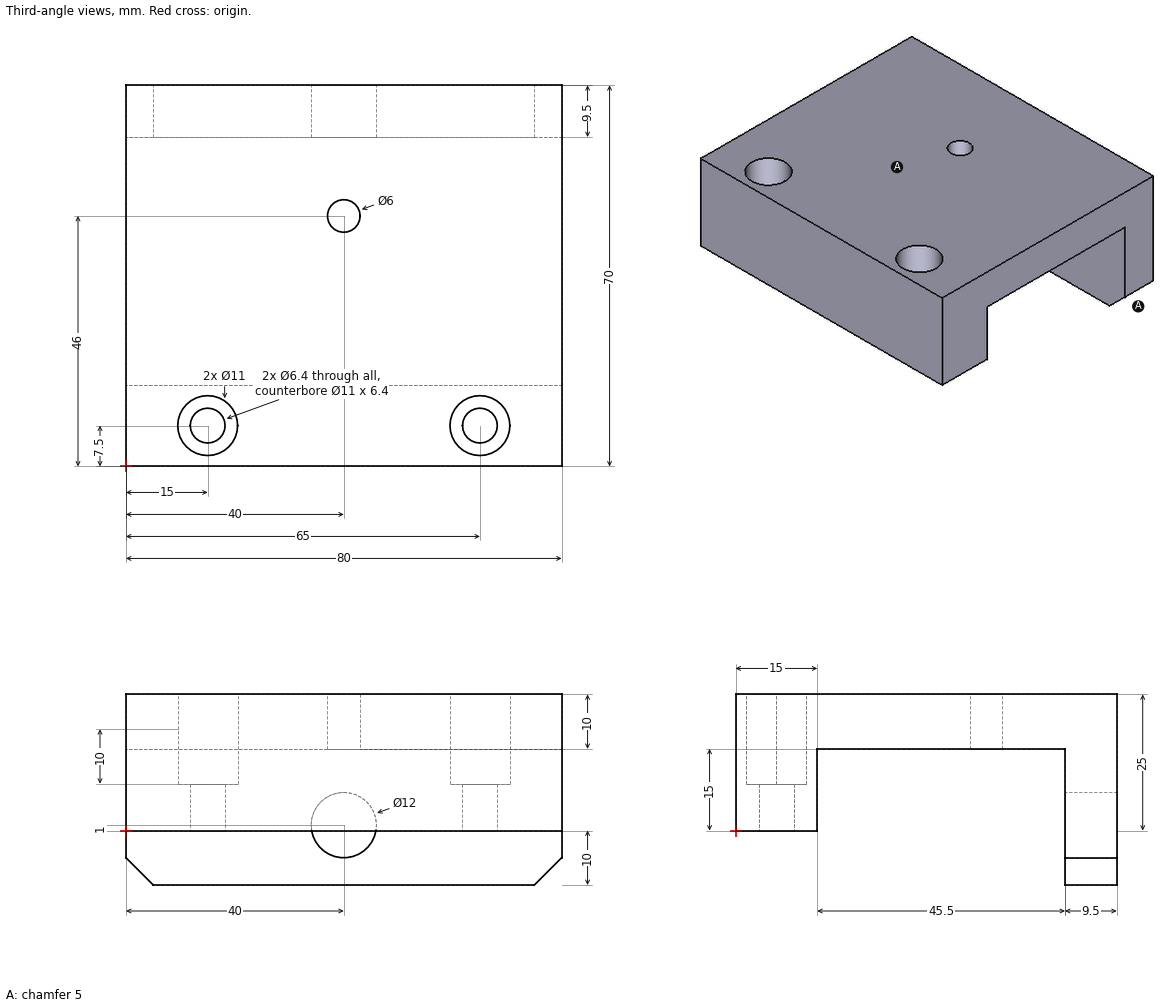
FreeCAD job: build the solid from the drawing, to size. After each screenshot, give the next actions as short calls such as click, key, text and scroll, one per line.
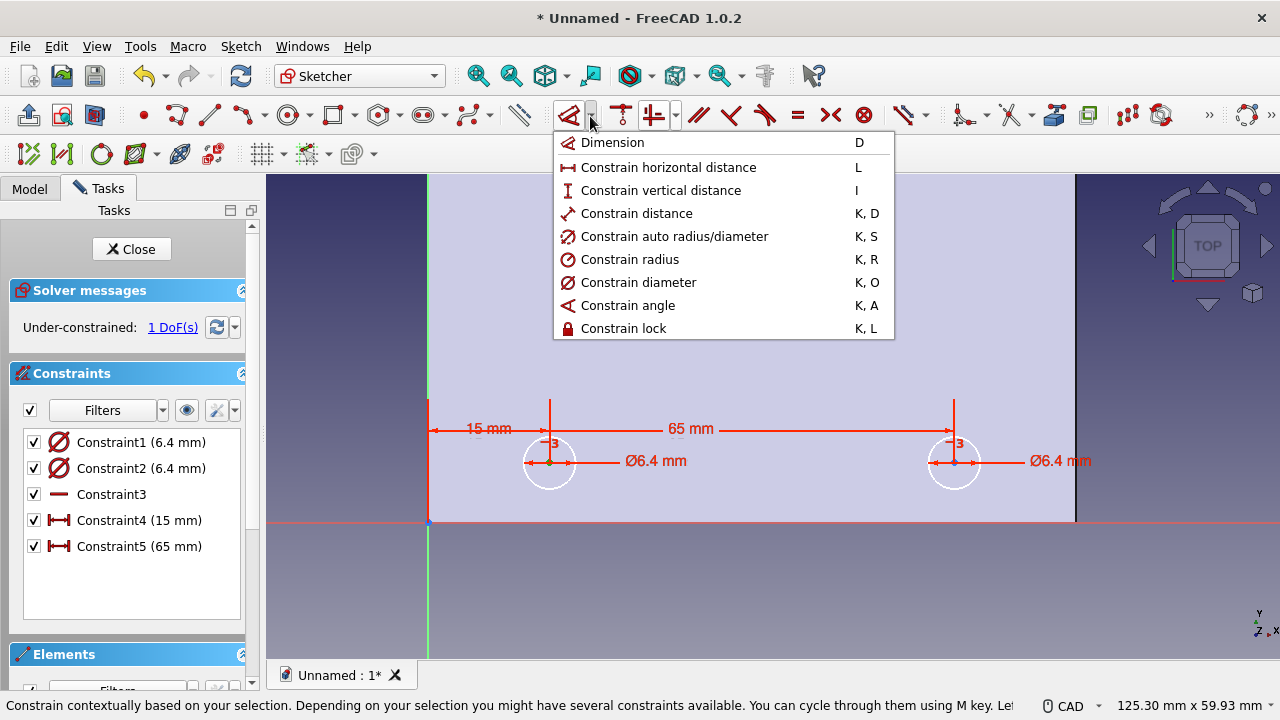
click(724, 190)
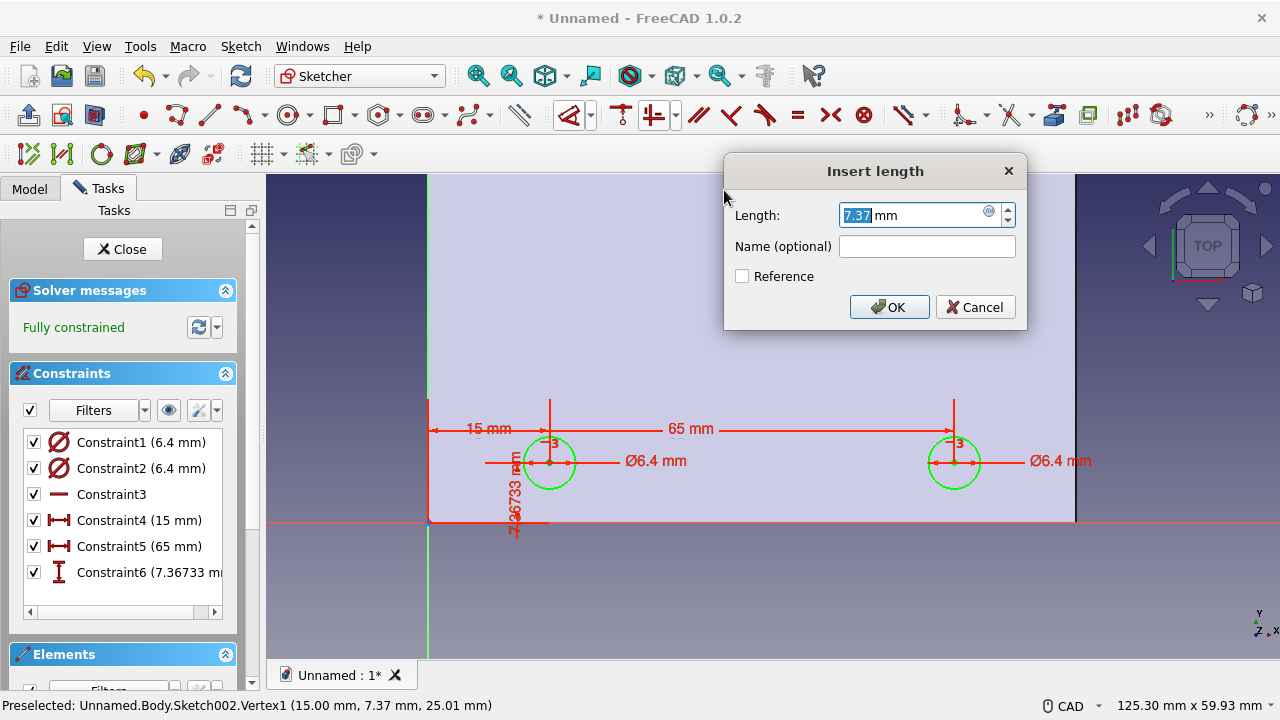
text(7.5)
key(Return)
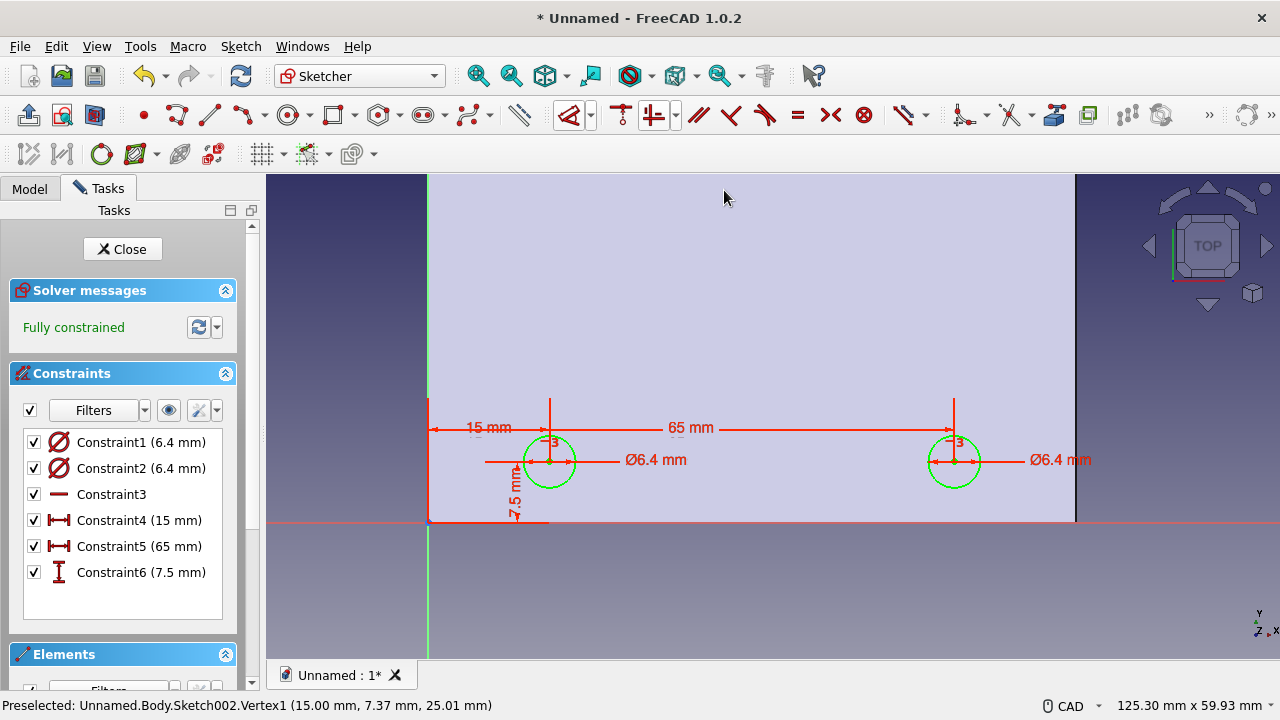
click(123, 249)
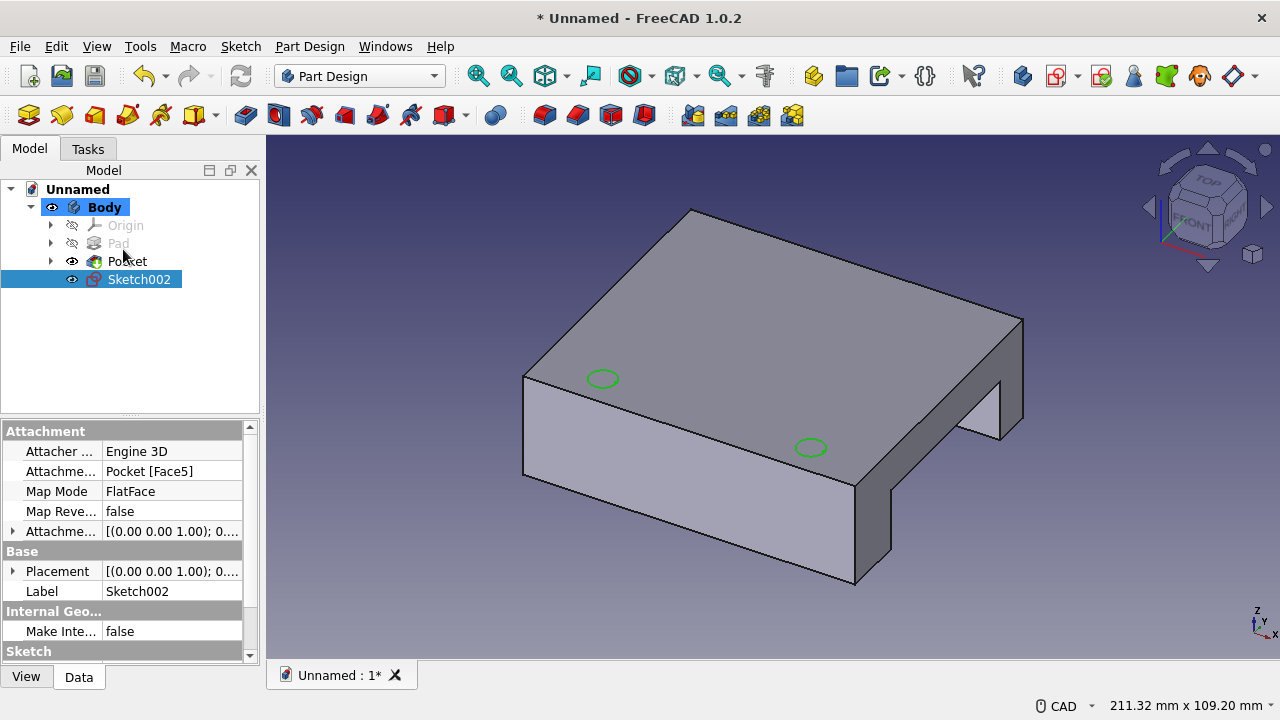
click(279, 116)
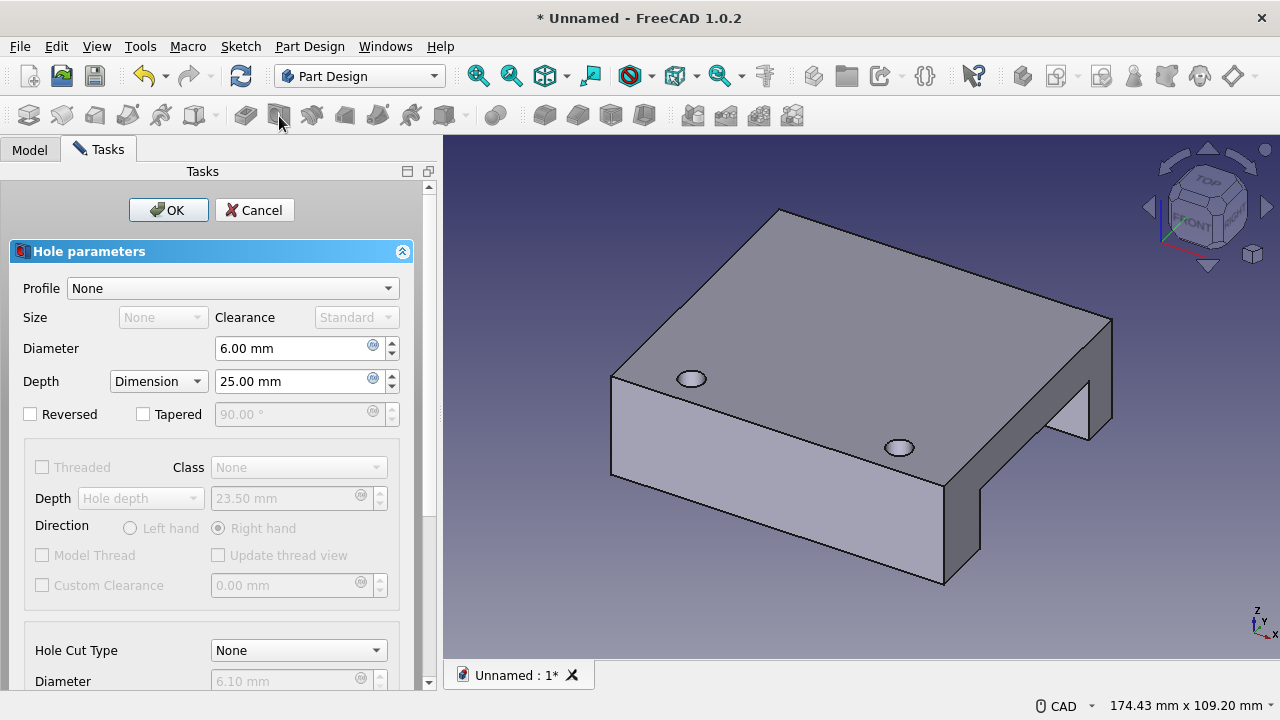
triple_click(300, 348)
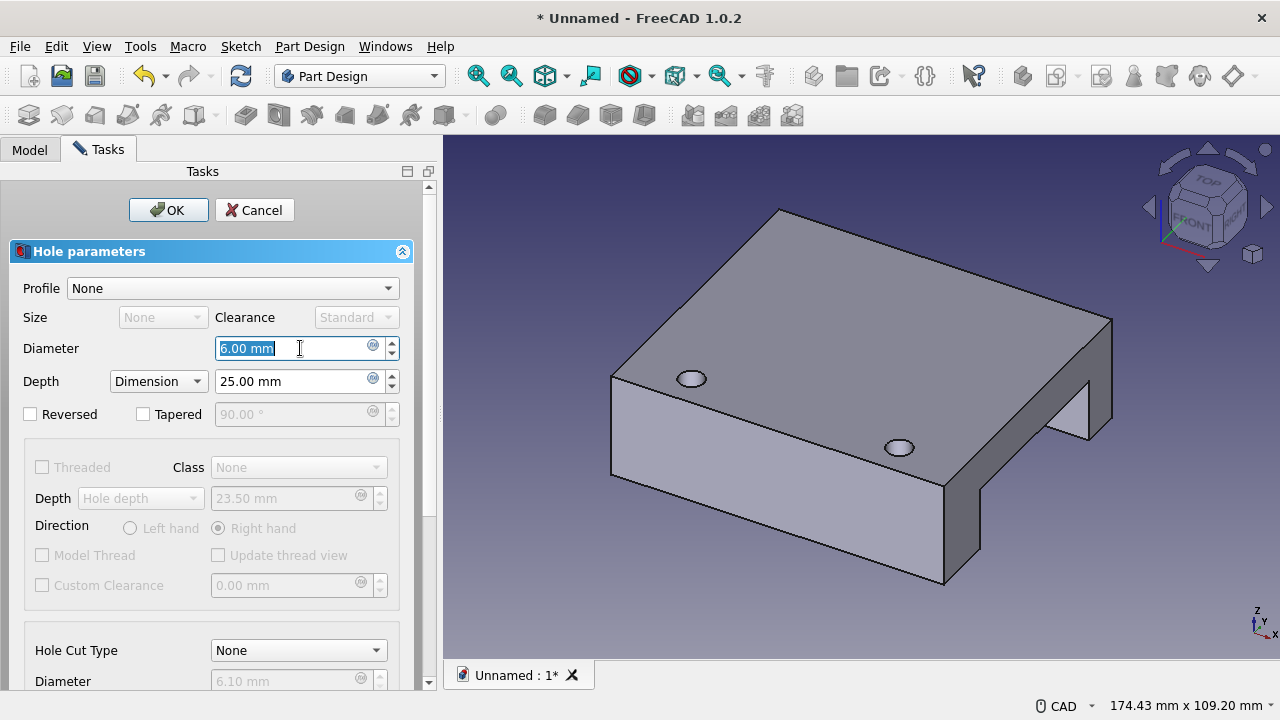
text(6.4)
key(Tab)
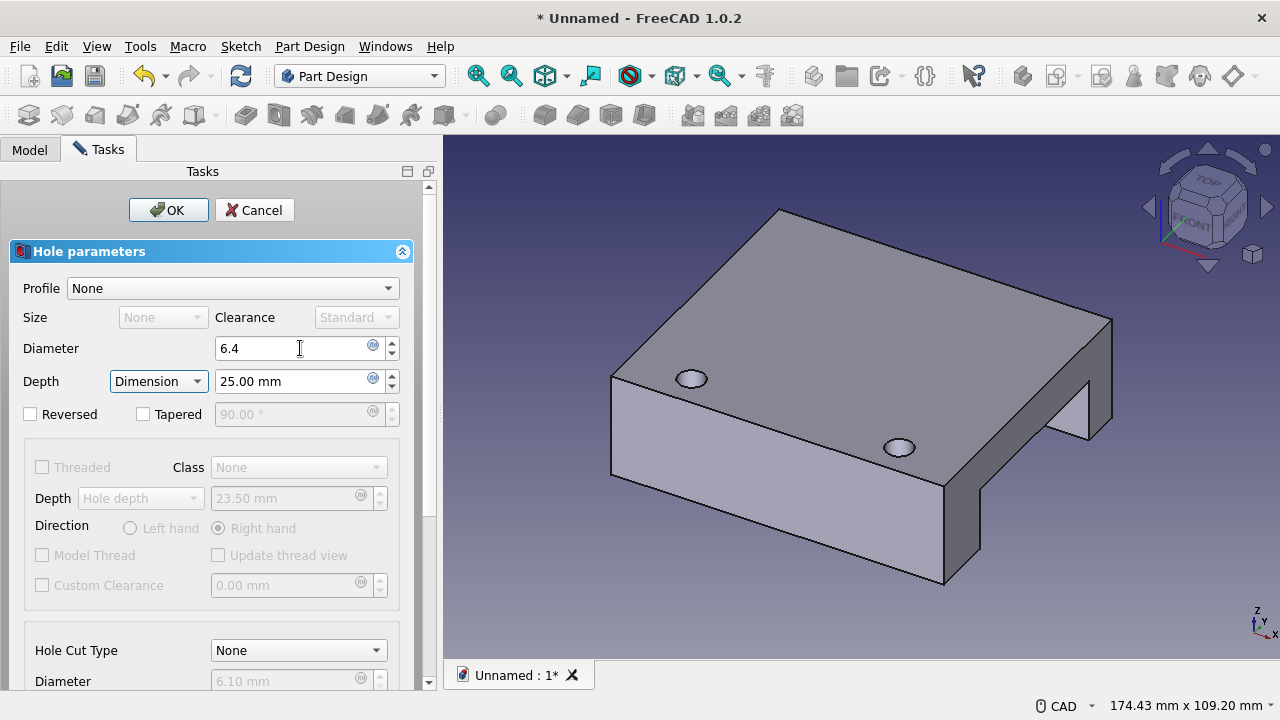
click(160, 382)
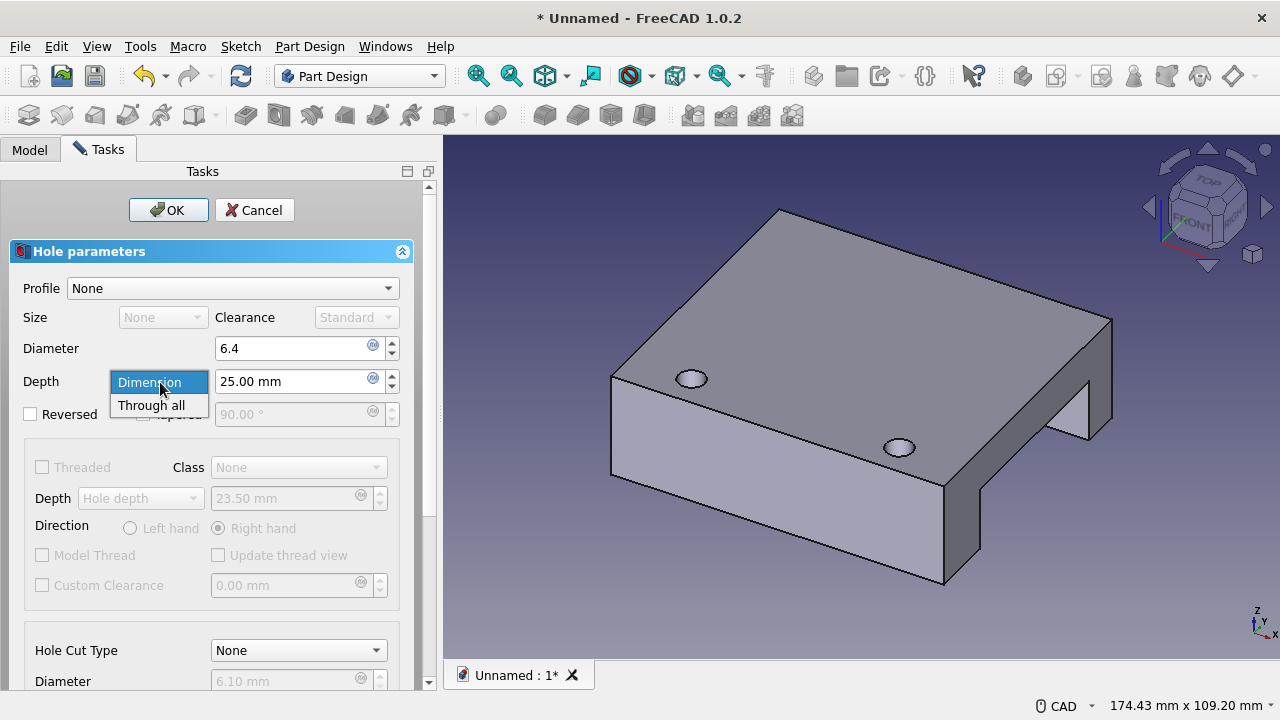
click(158, 406)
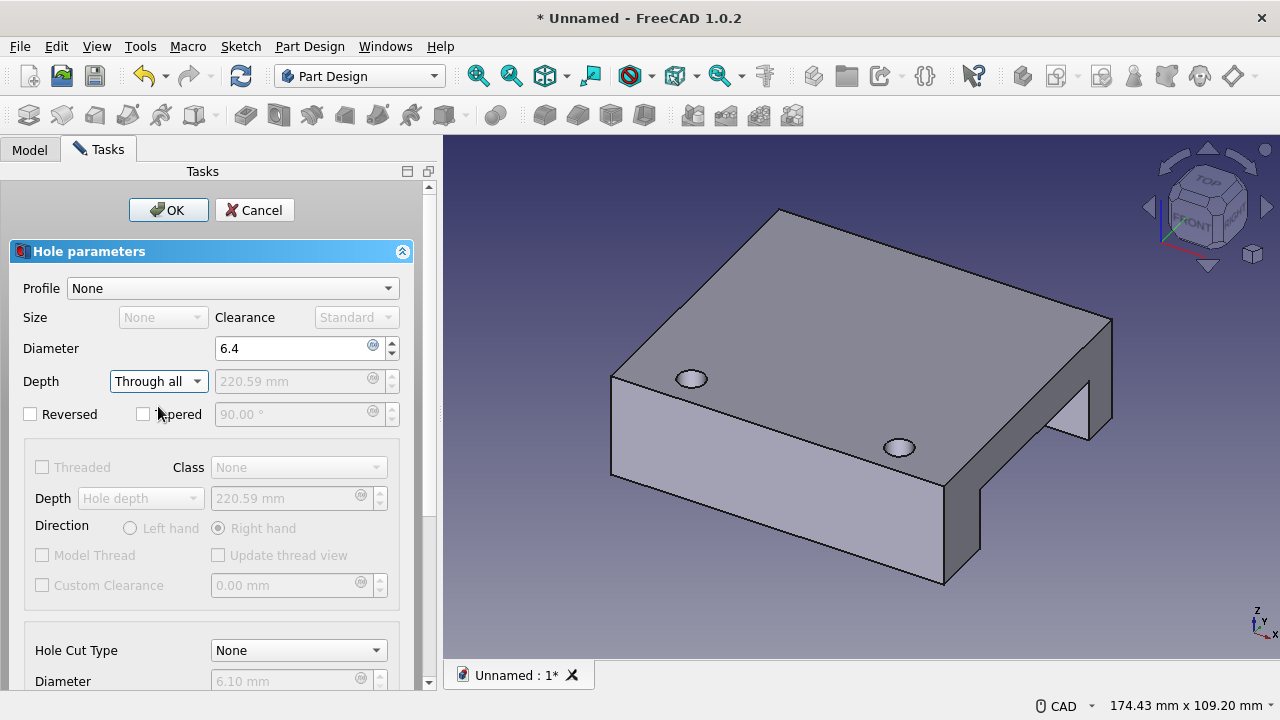
click(300, 650)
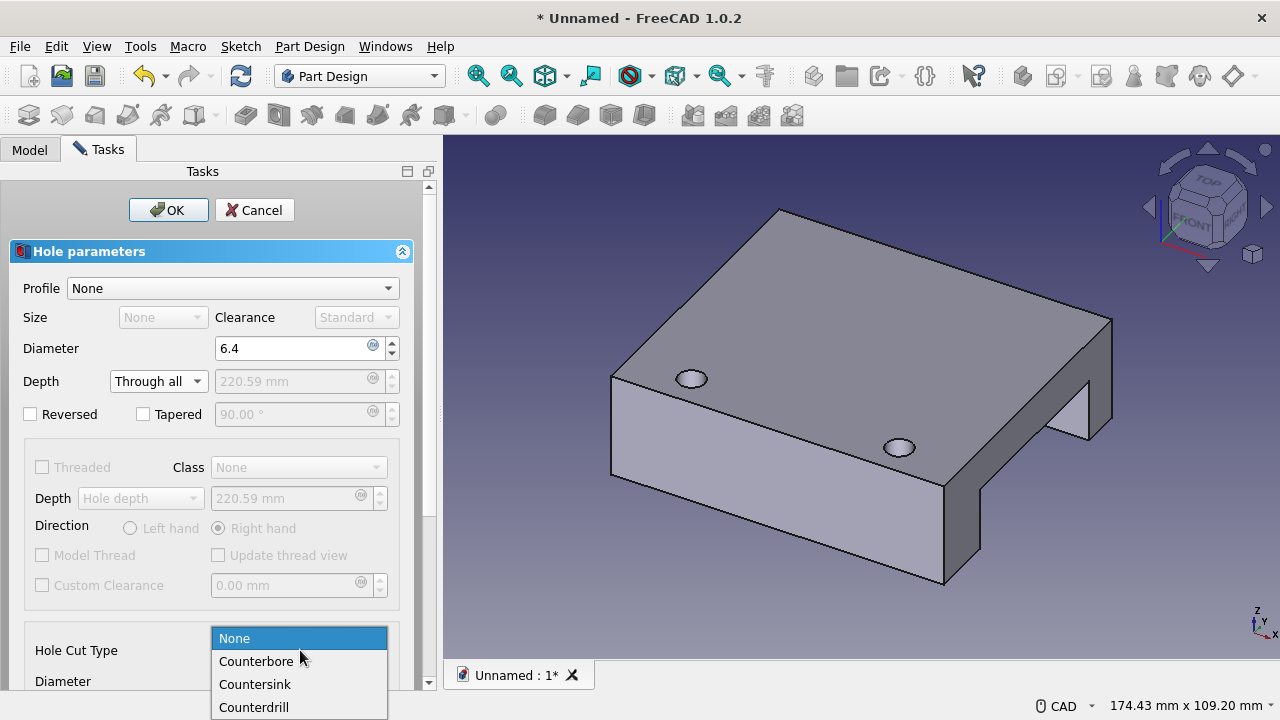
click(298, 662)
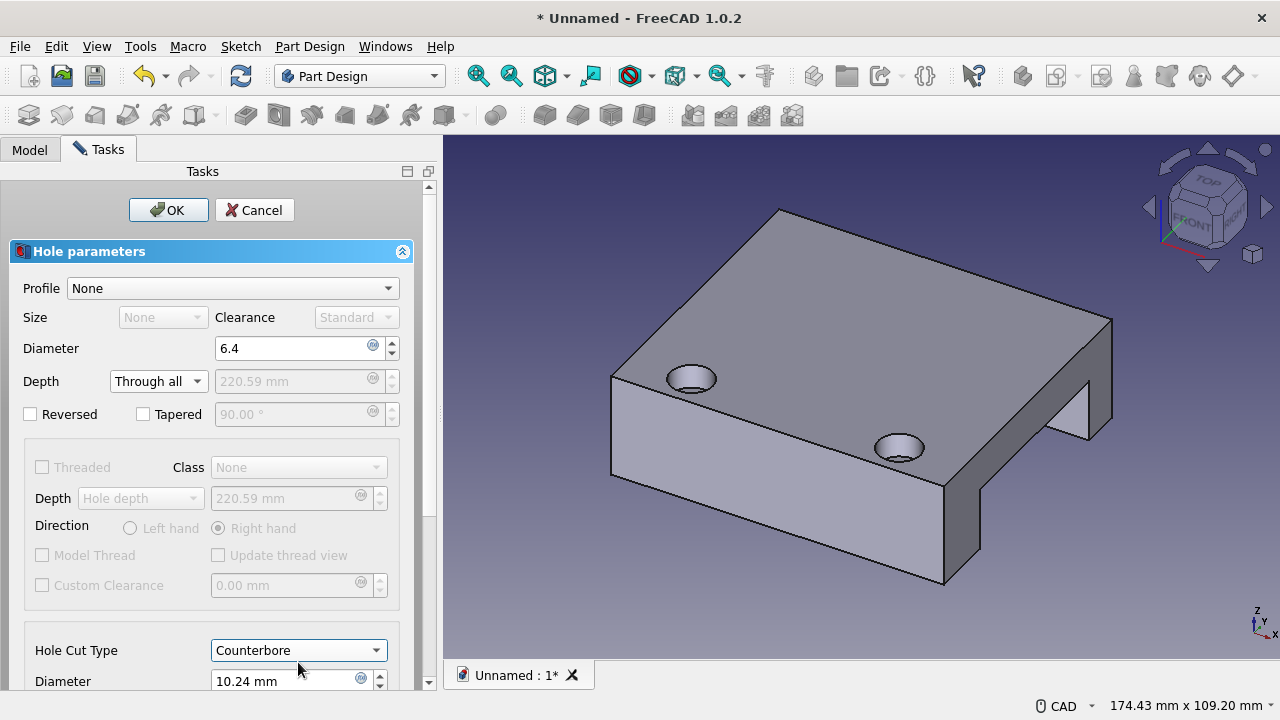
scroll(429, 436, down, 2)